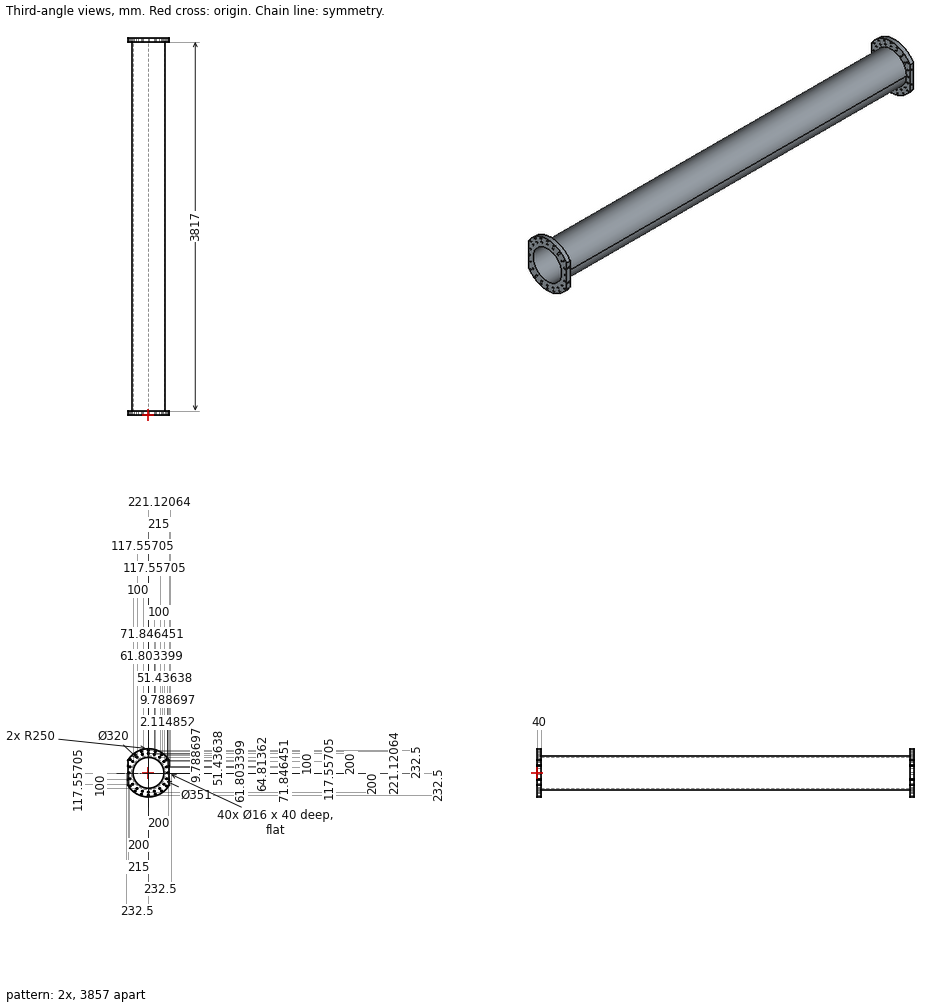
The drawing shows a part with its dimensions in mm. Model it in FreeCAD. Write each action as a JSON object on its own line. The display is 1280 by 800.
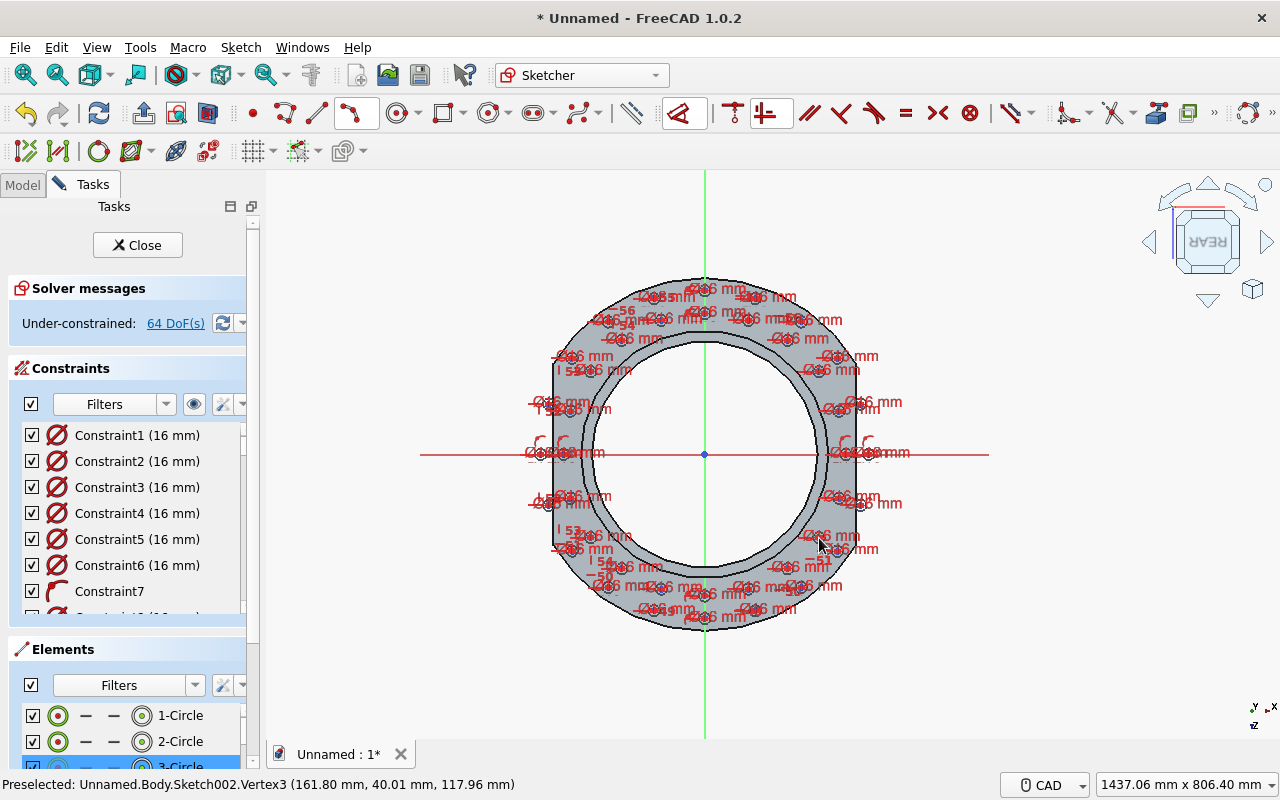
{"action": "left_click", "coordinate": [819, 372]}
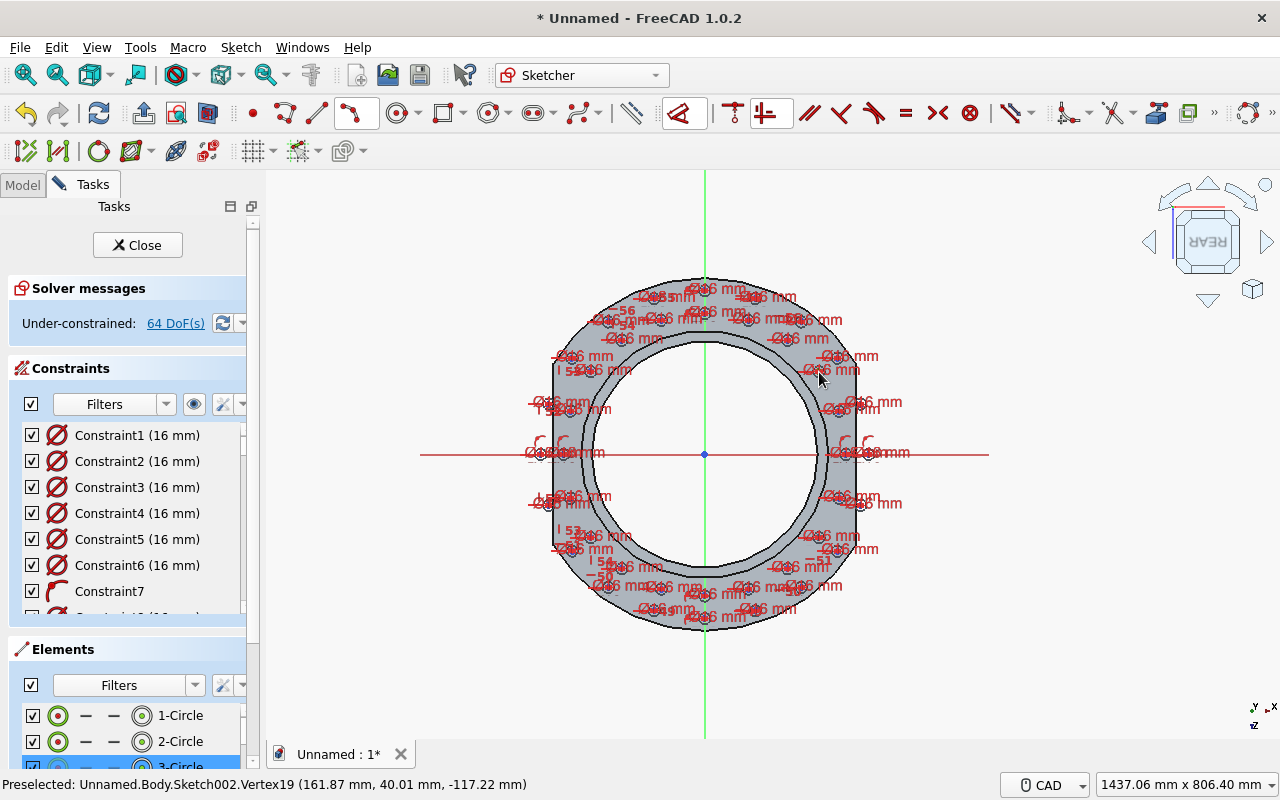
{"action": "key", "text": "v"}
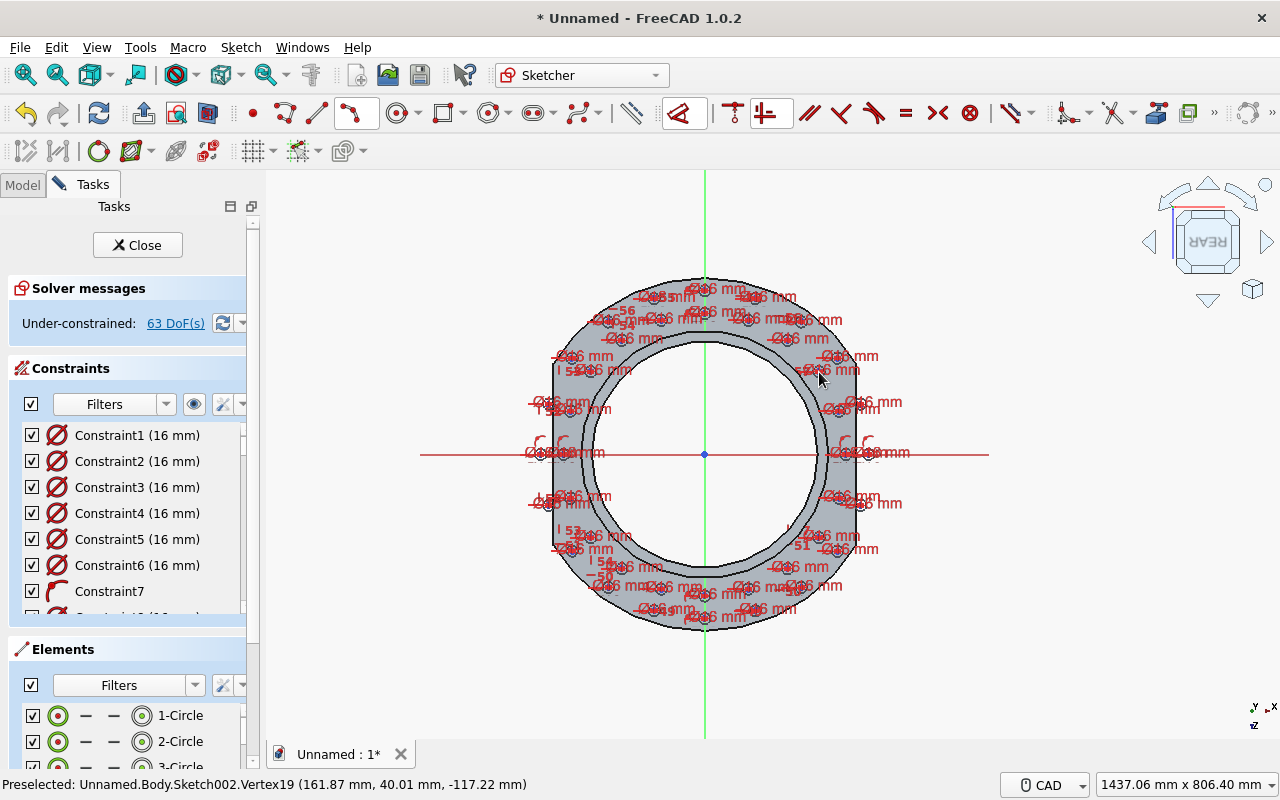
{"action": "left_click", "coordinate": [839, 498]}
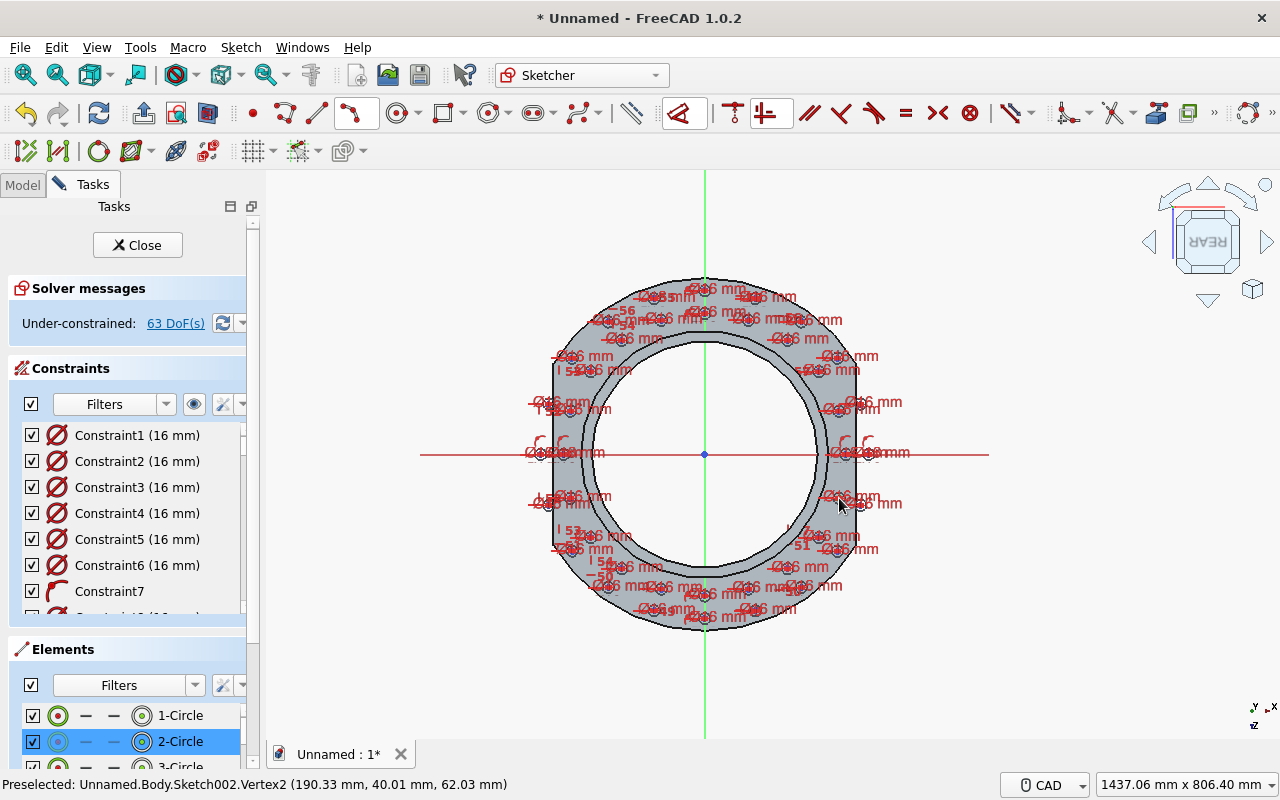
{"action": "left_click", "coordinate": [839, 411]}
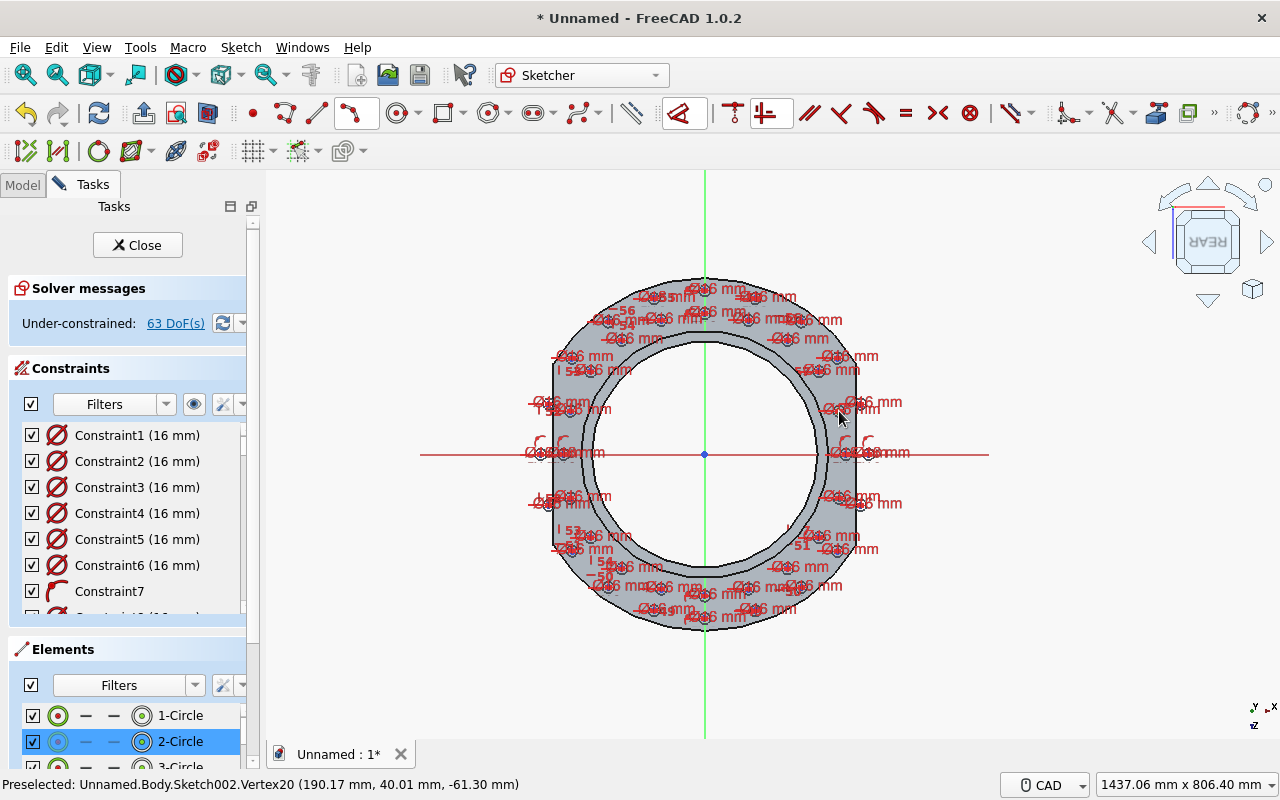
{"action": "left_click", "coordinate": [788, 114]}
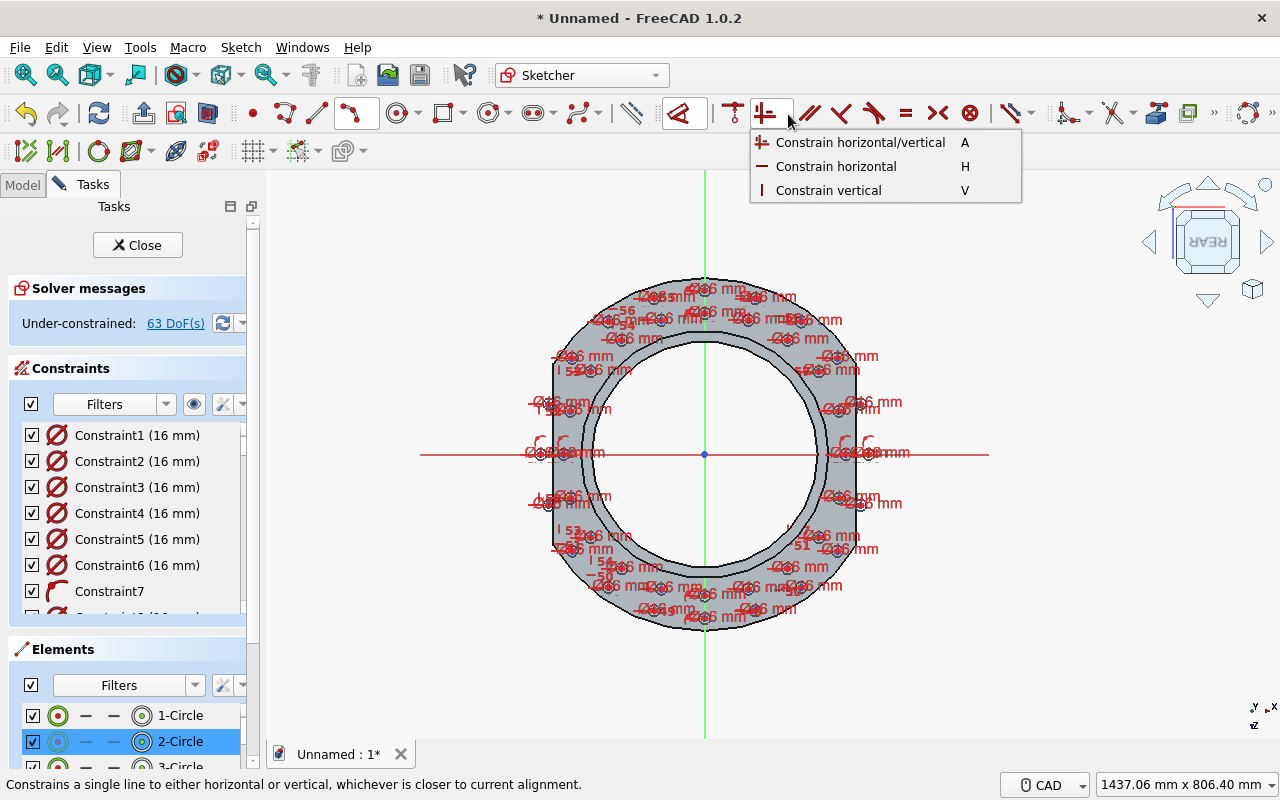
{"action": "left_click", "coordinate": [886, 190]}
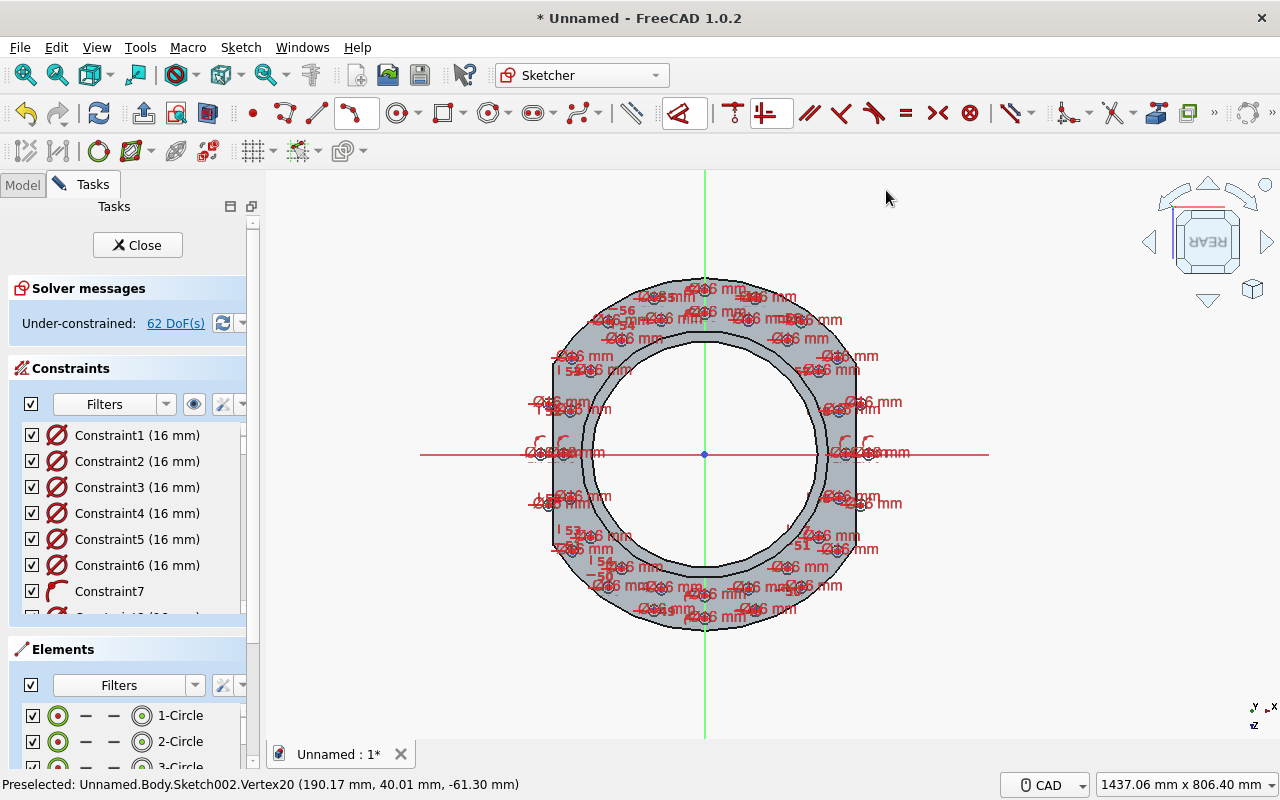
{"action": "left_click", "coordinate": [839, 498]}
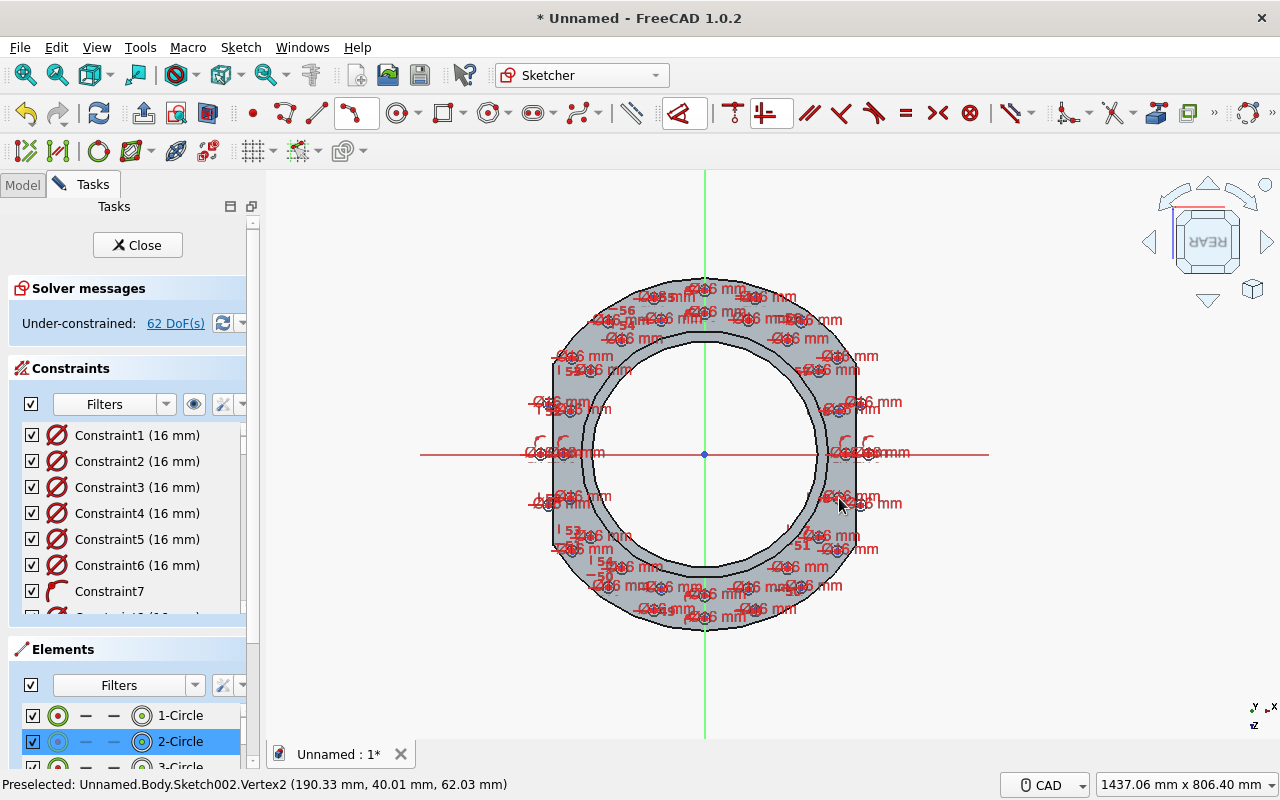
{"action": "left_click", "coordinate": [570, 498]}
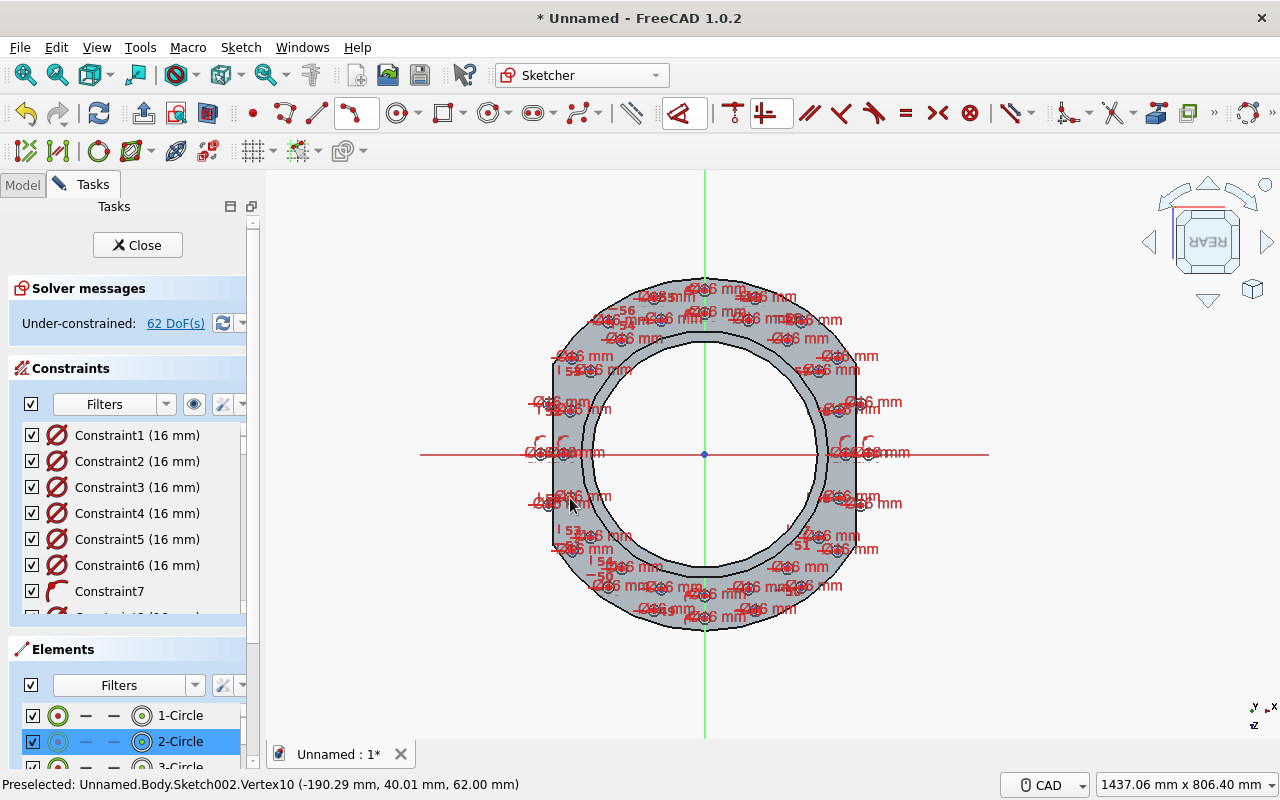
{"action": "left_click", "coordinate": [705, 674]}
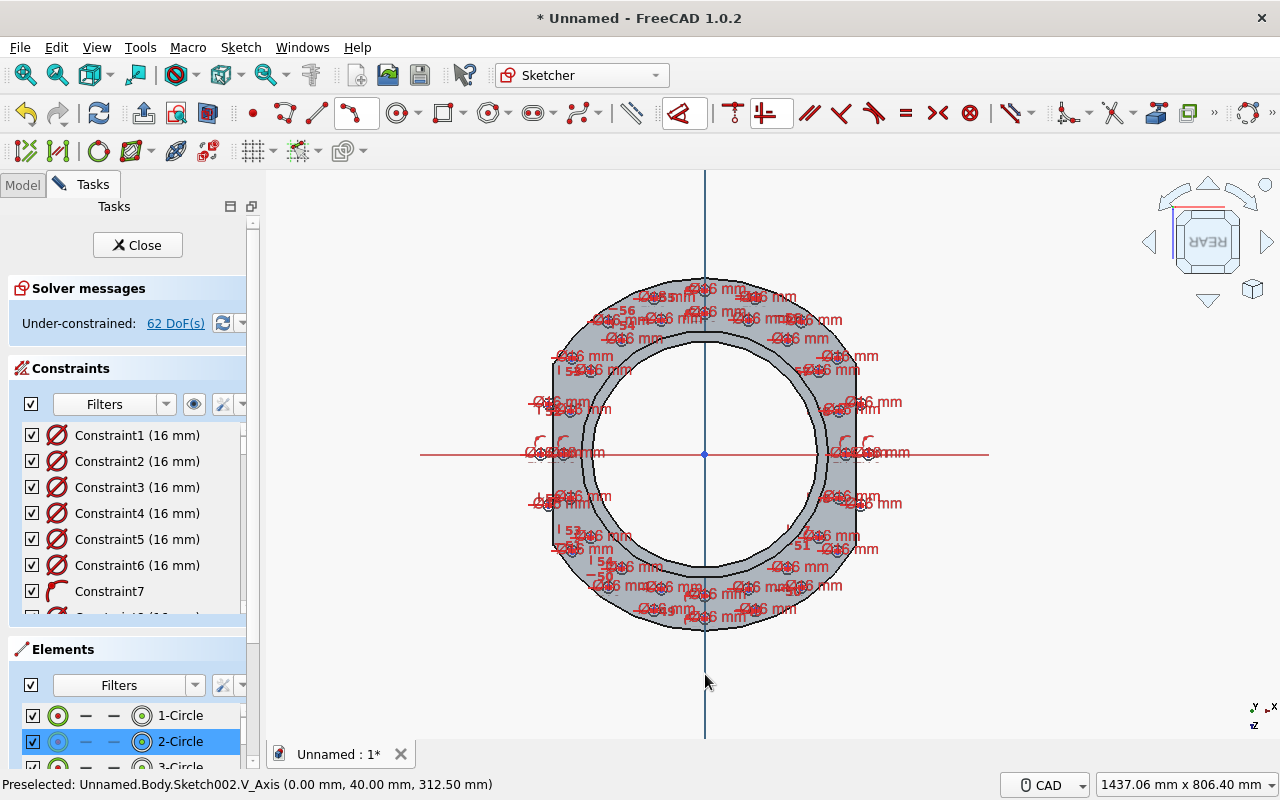
{"action": "left_click", "coordinate": [938, 114]}